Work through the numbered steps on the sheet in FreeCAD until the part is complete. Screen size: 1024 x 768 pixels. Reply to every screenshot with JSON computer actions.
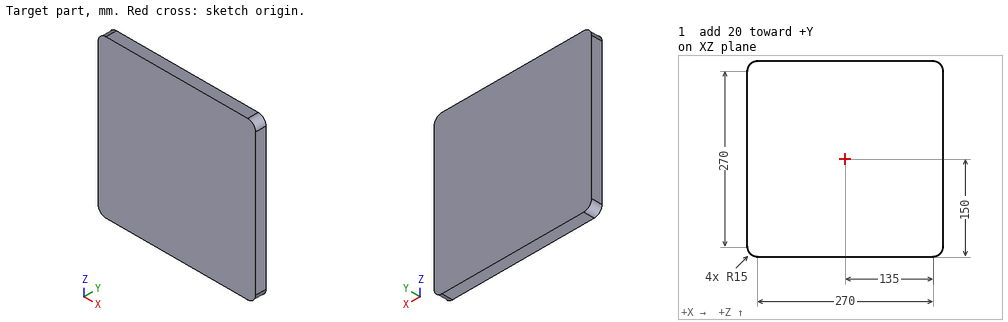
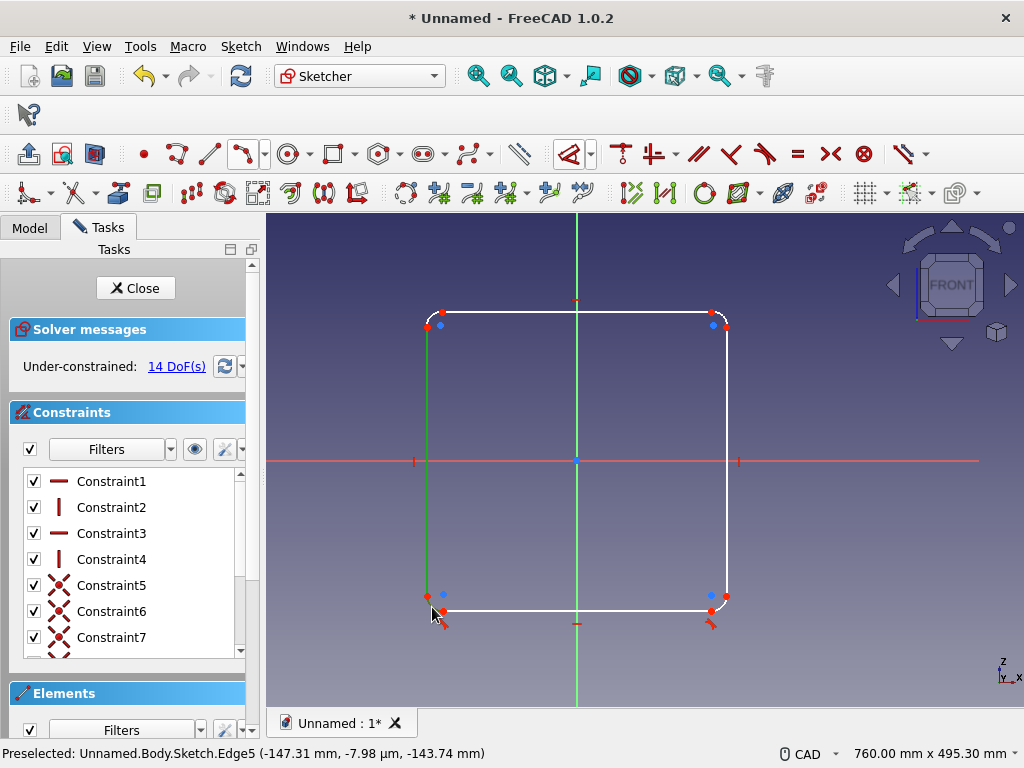
{"action": "left_click", "coordinate": [765, 154]}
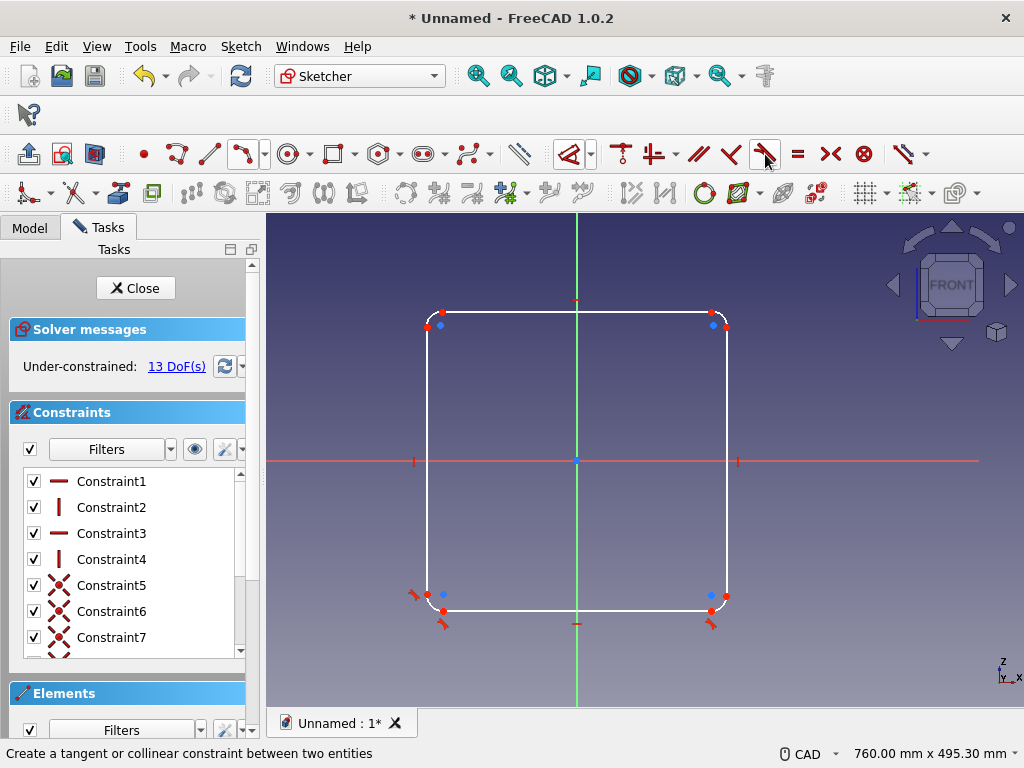
{"action": "left_click", "coordinate": [427, 515]}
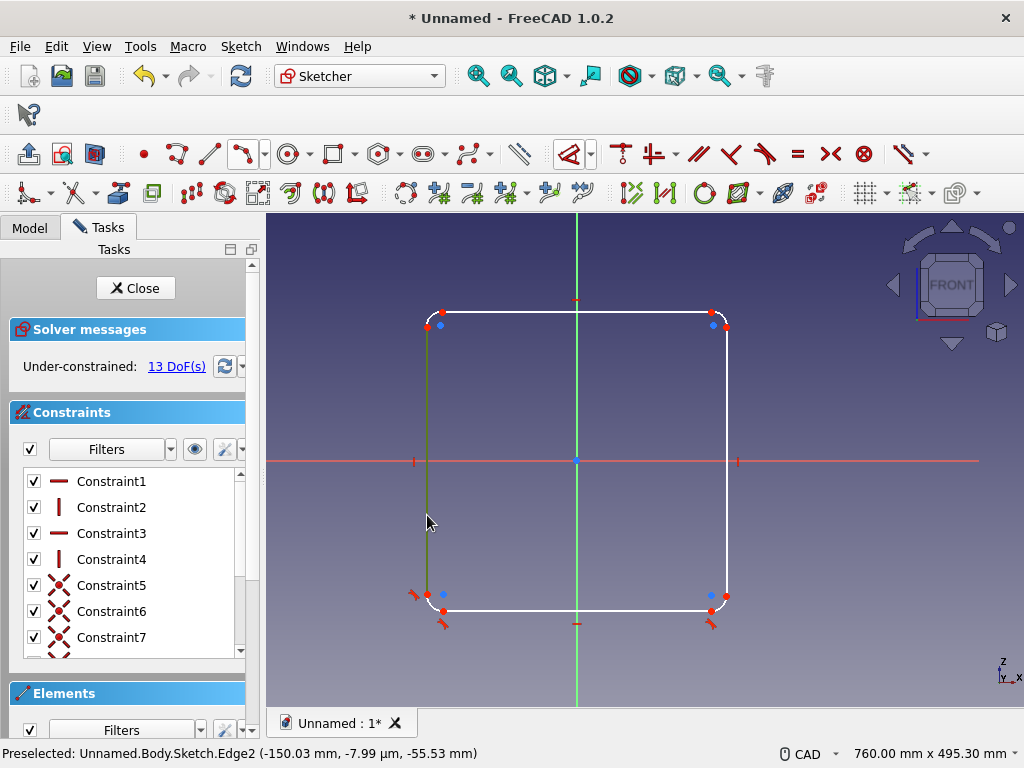
{"action": "left_click", "coordinate": [431, 316]}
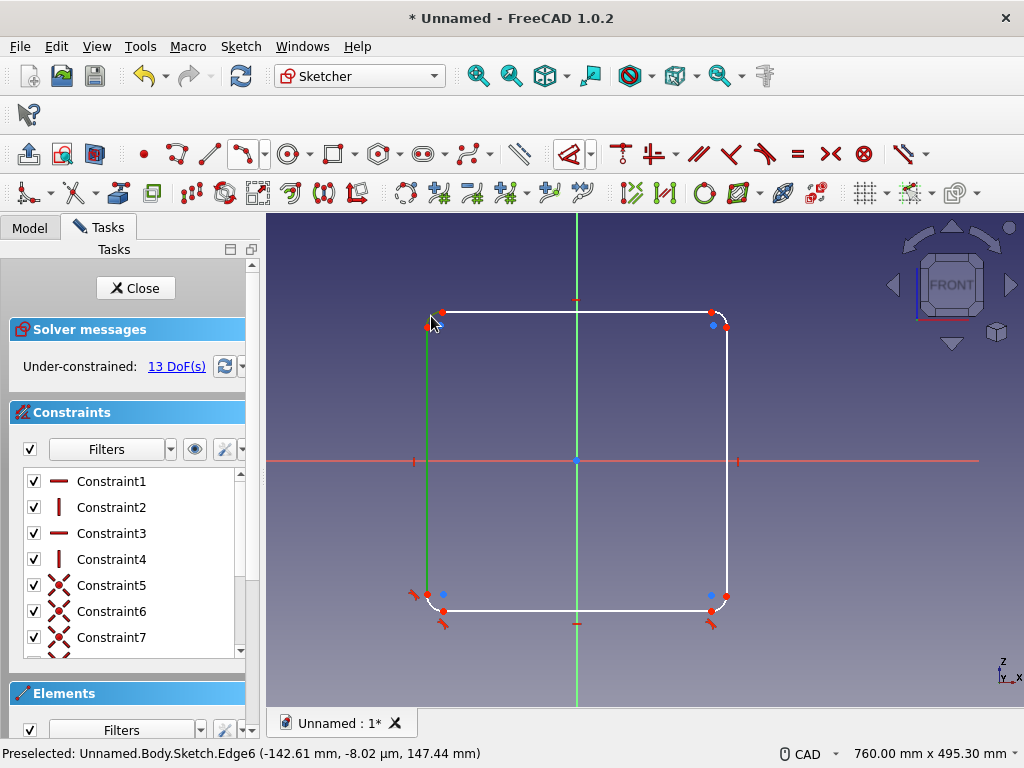
{"action": "left_click", "coordinate": [765, 154]}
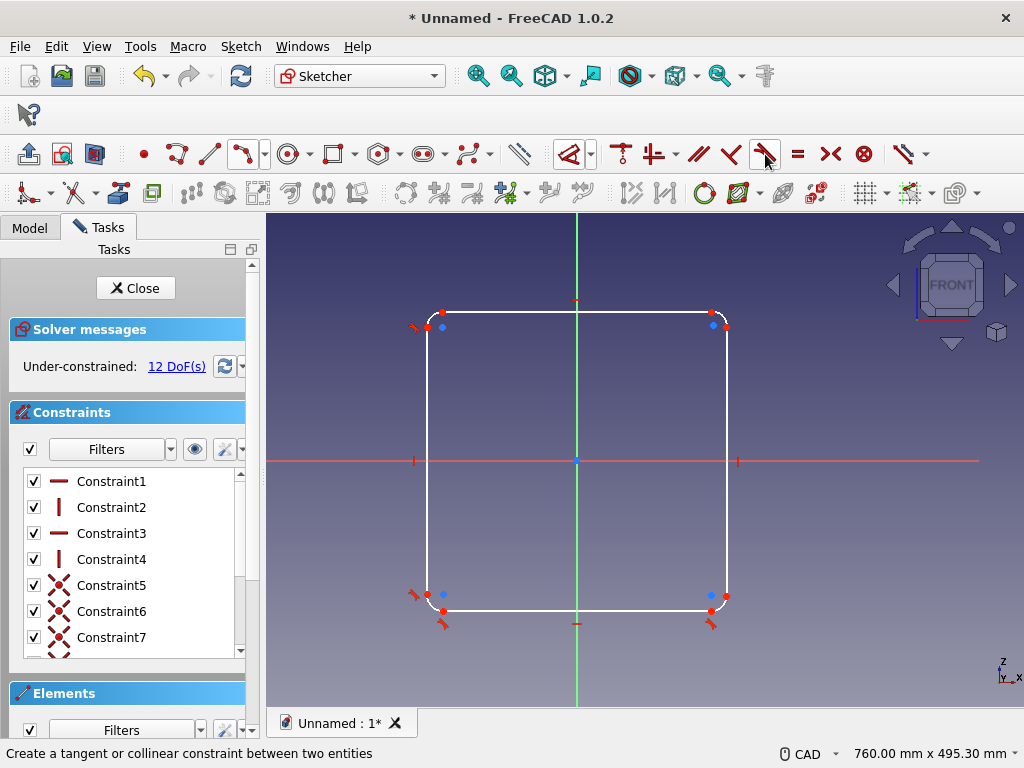
{"action": "left_click", "coordinate": [523, 312]}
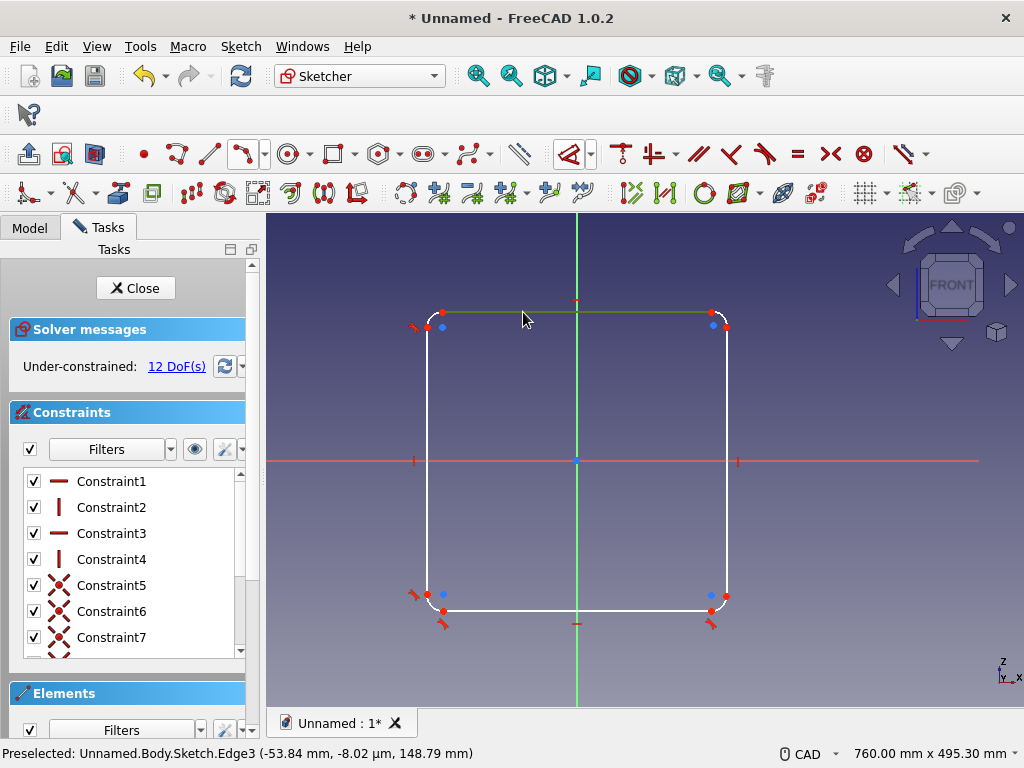
{"action": "left_click", "coordinate": [431, 317]}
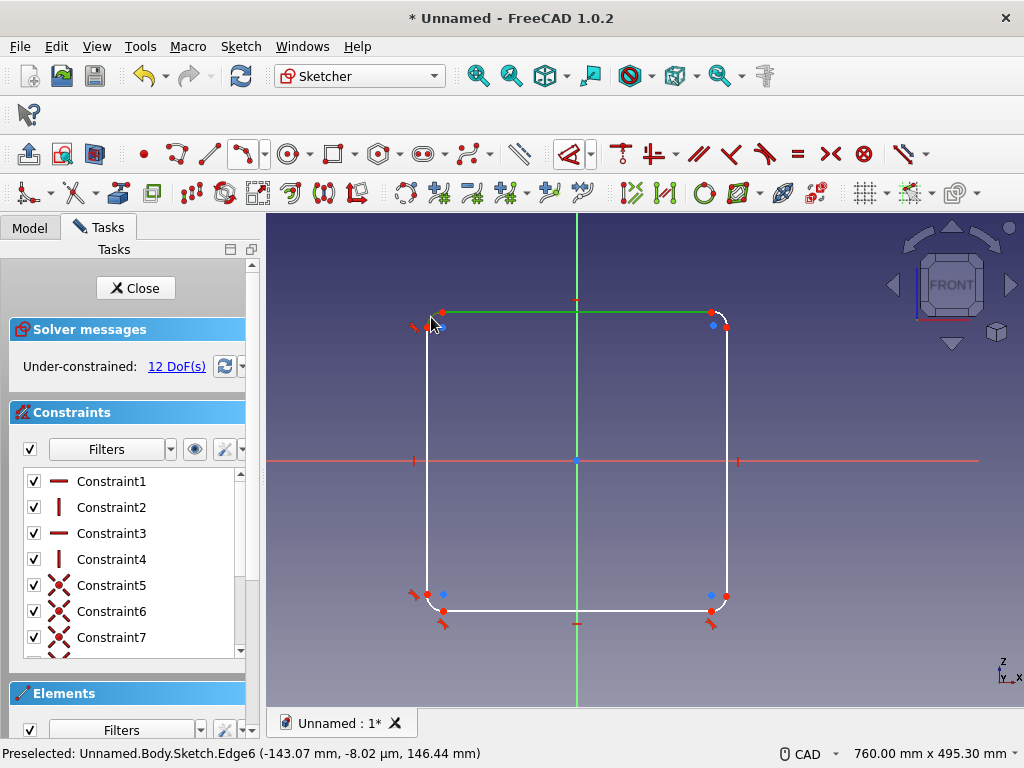
{"action": "key", "text": "t"}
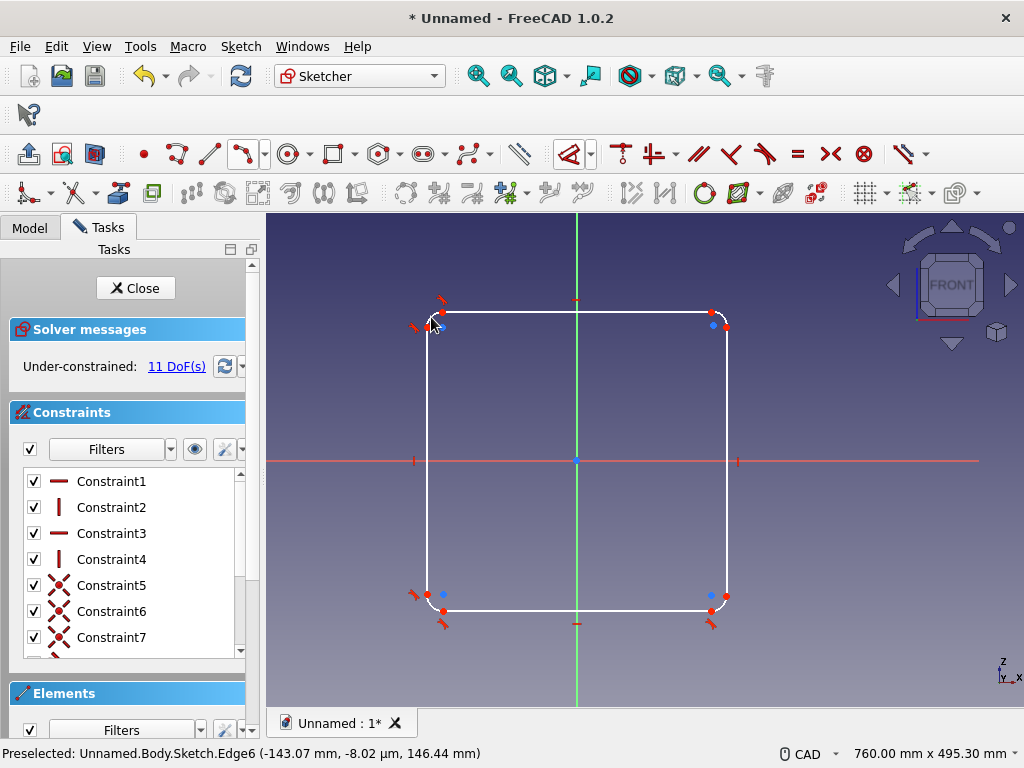
{"action": "left_click", "coordinate": [523, 312]}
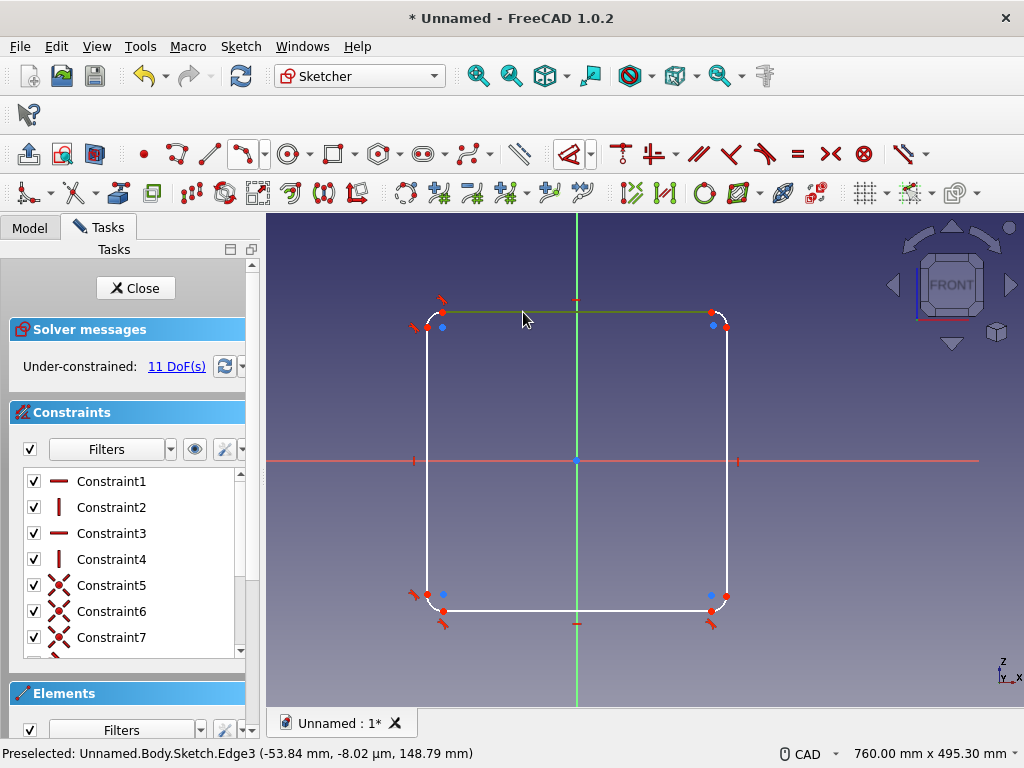
{"action": "left_click", "coordinate": [723, 316]}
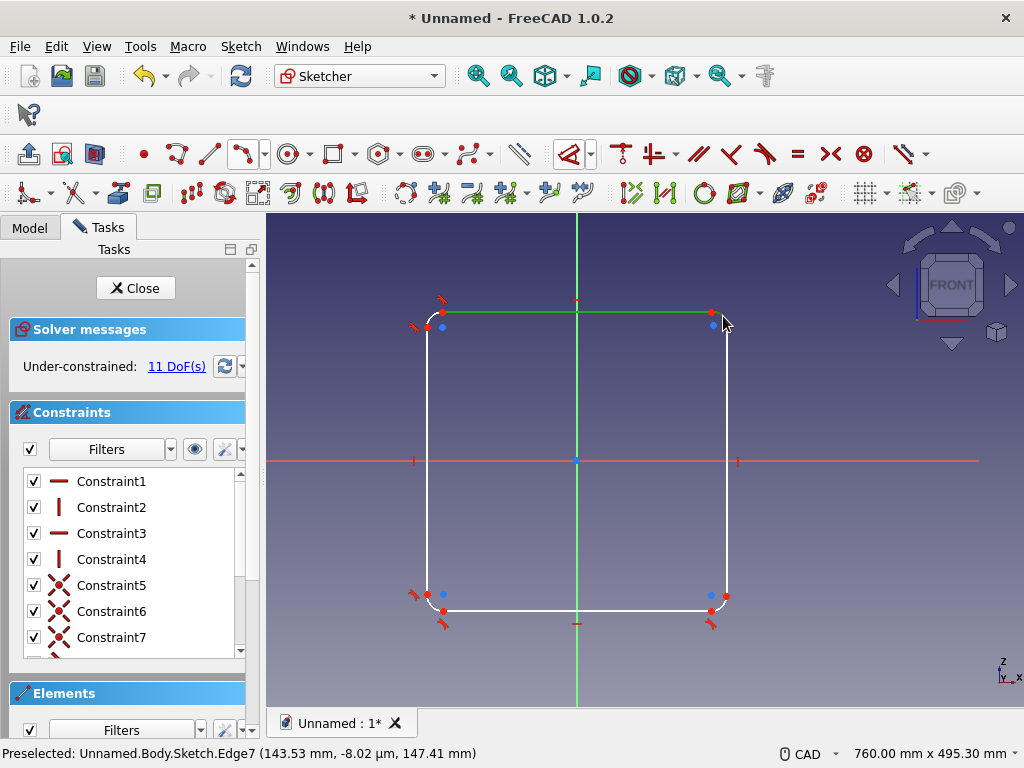
{"action": "left_click", "coordinate": [765, 154]}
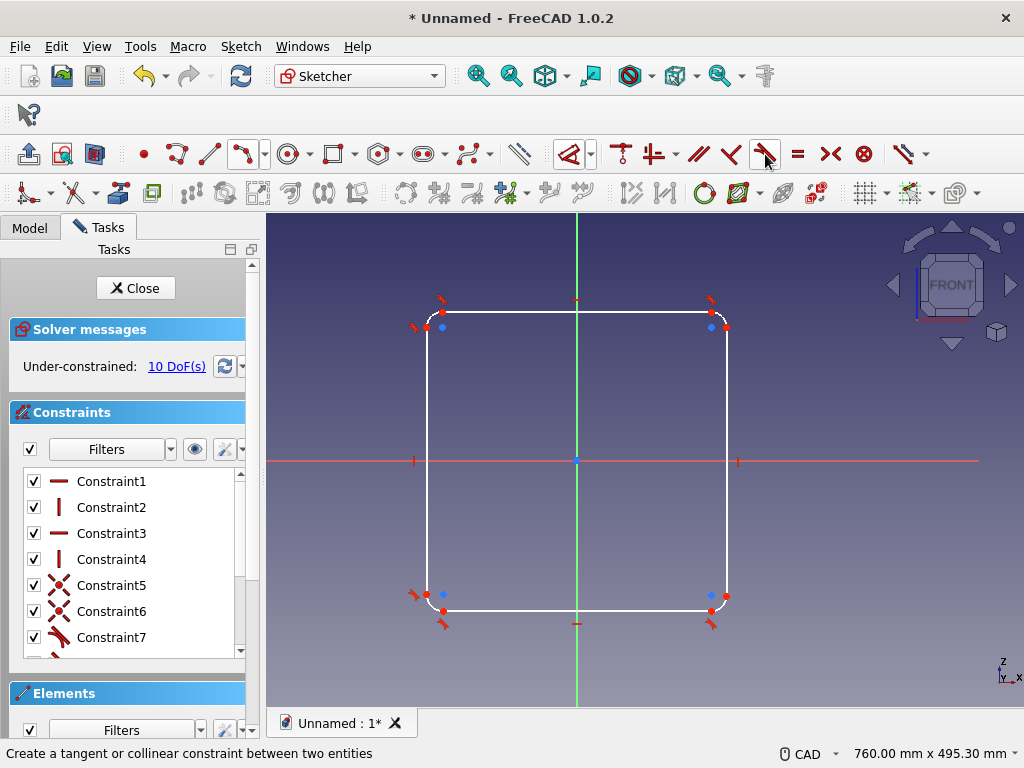
{"action": "left_click", "coordinate": [727, 408]}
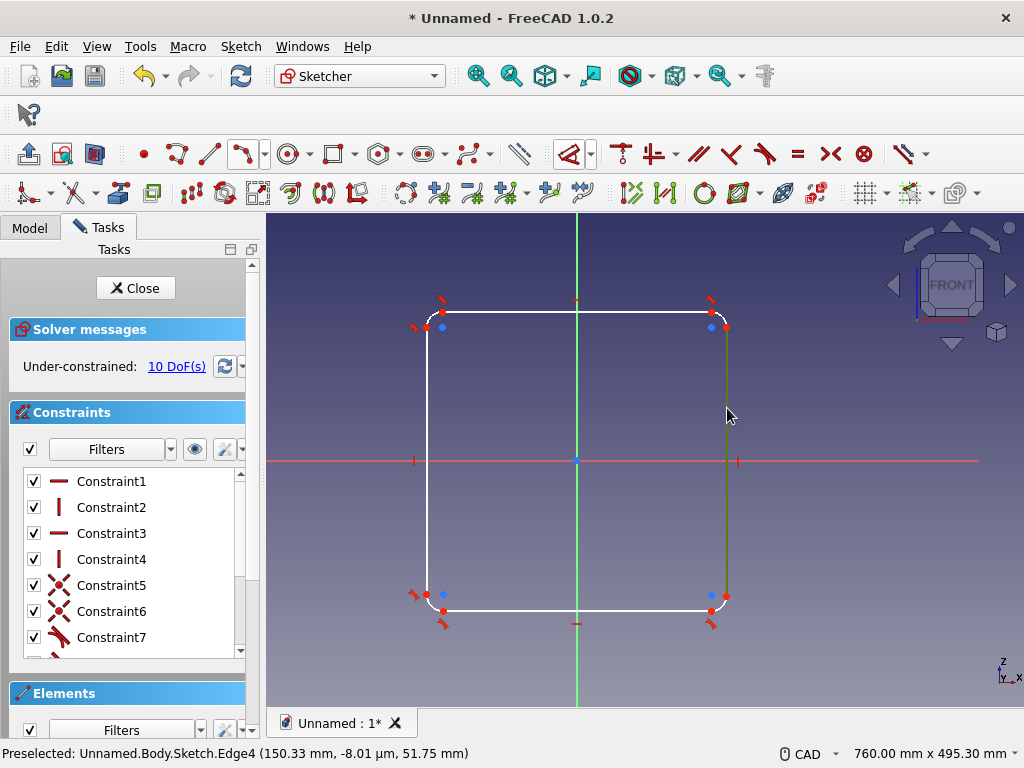
{"action": "left_click", "coordinate": [722, 316]}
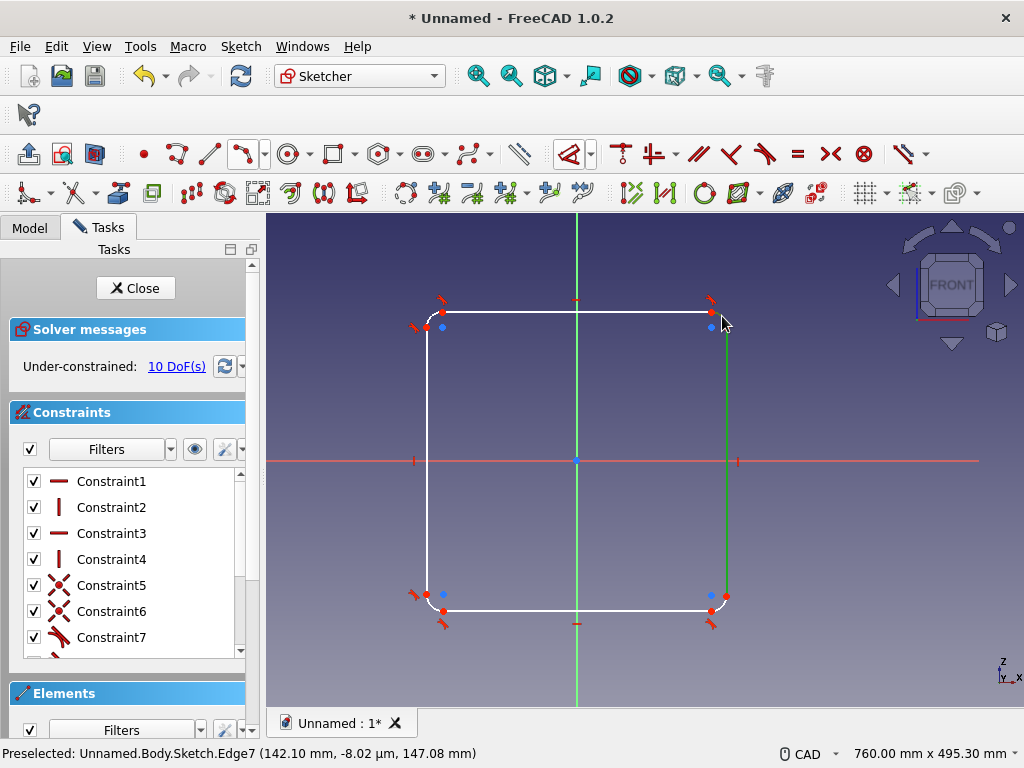
{"action": "left_click", "coordinate": [765, 154]}